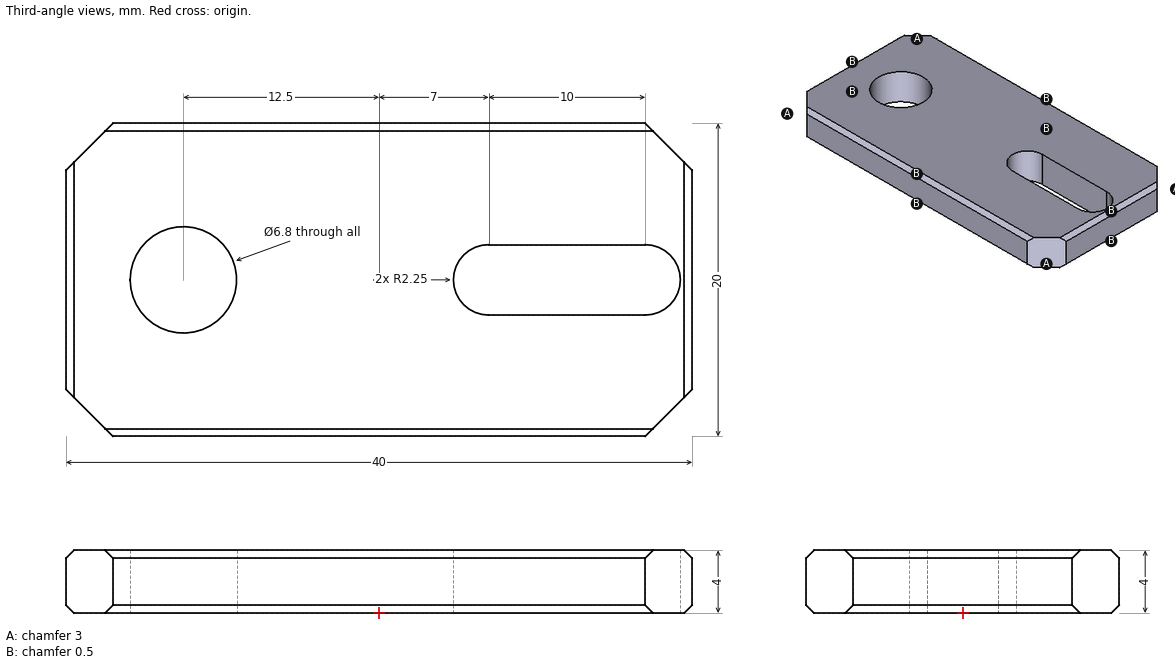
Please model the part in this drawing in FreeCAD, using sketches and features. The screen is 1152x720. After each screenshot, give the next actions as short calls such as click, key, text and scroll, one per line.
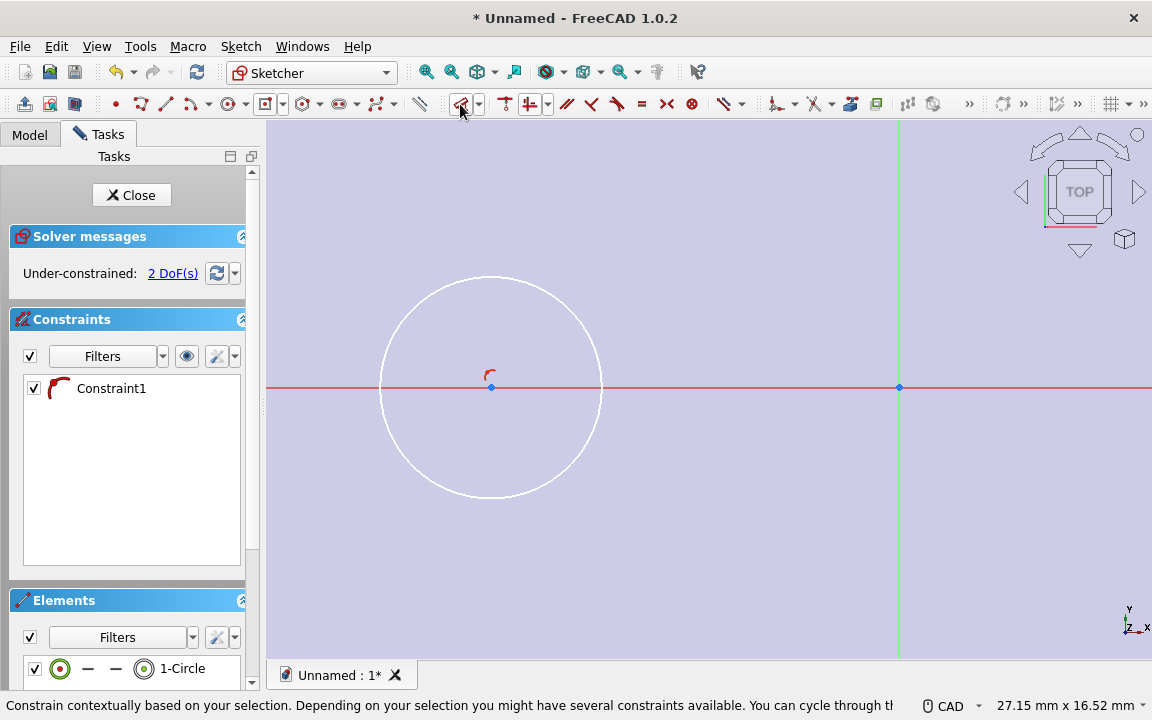
click(569, 309)
click(592, 286)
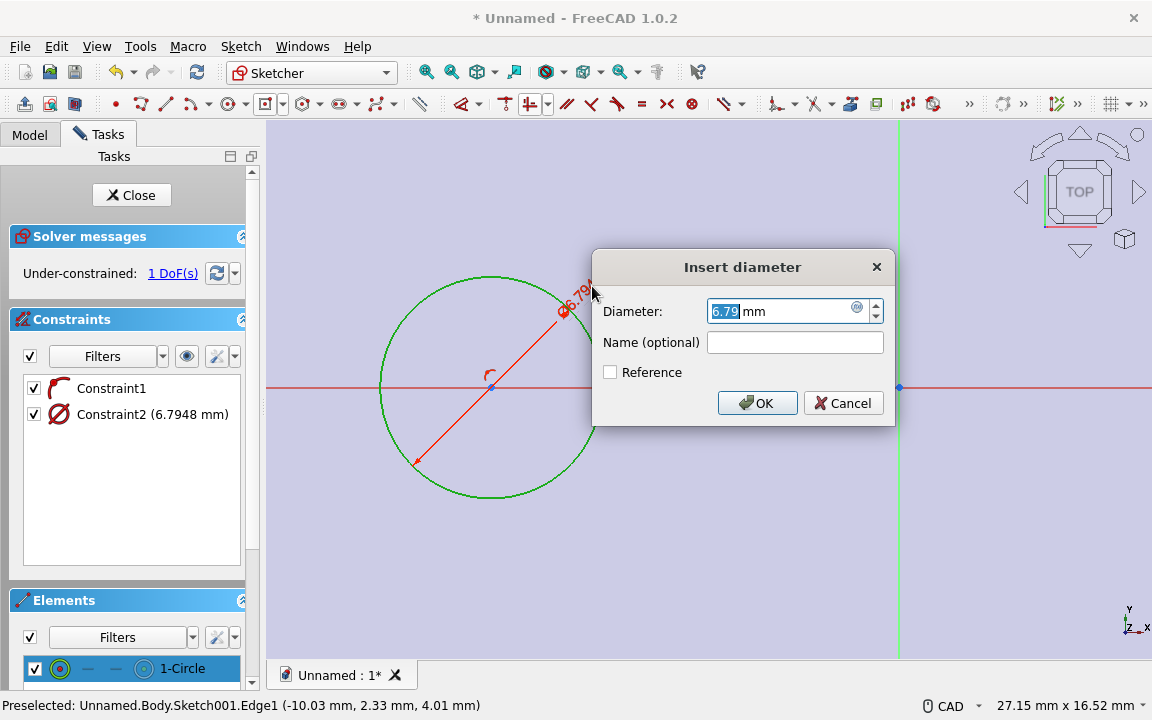
text(6.8)
key(Return)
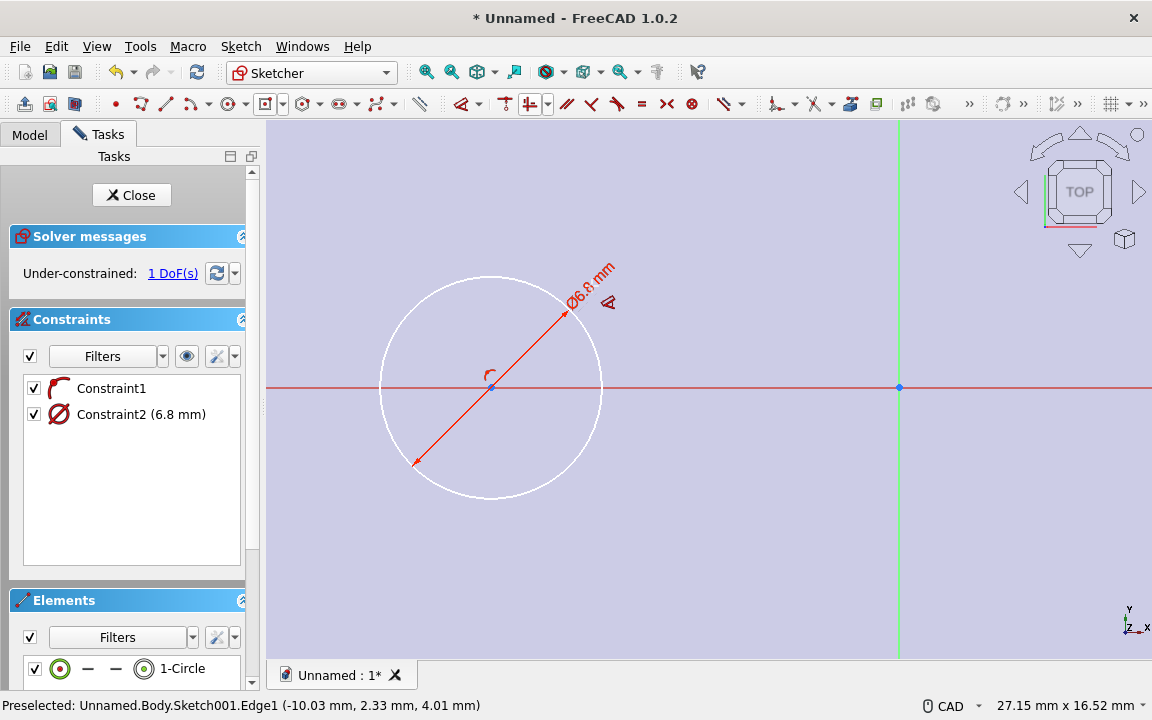
click(491, 388)
click(695, 422)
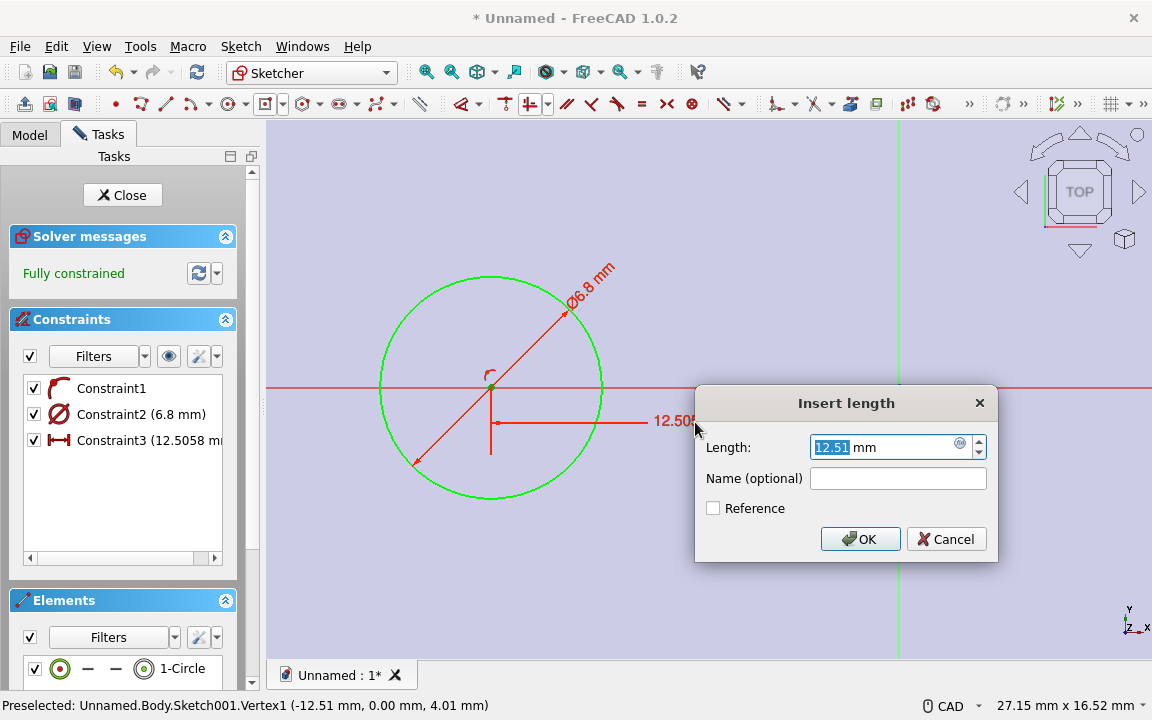
text(12.5)
key(Return)
key(Escape)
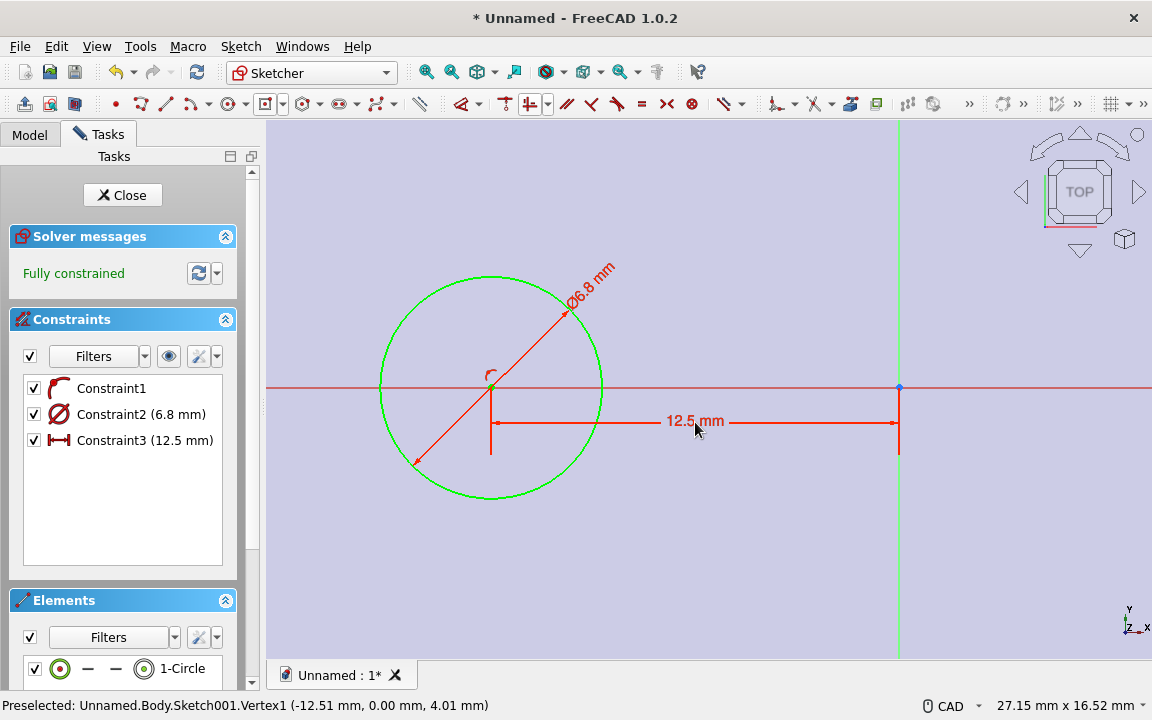
click(123, 195)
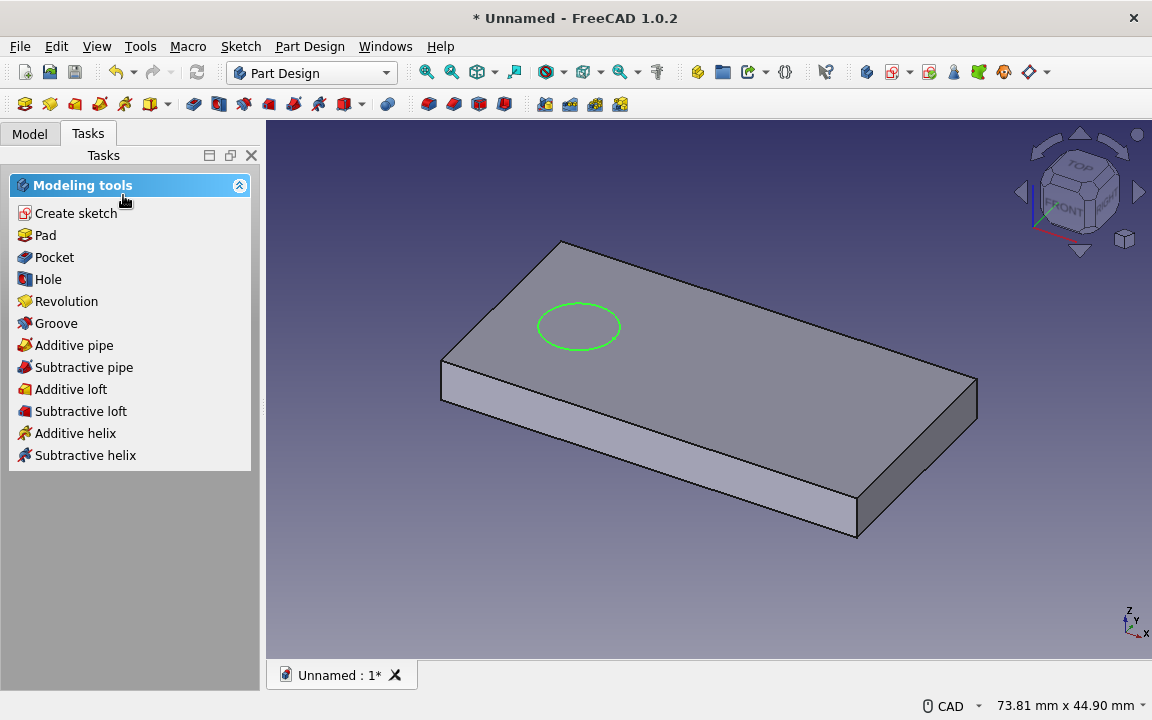
click(219, 104)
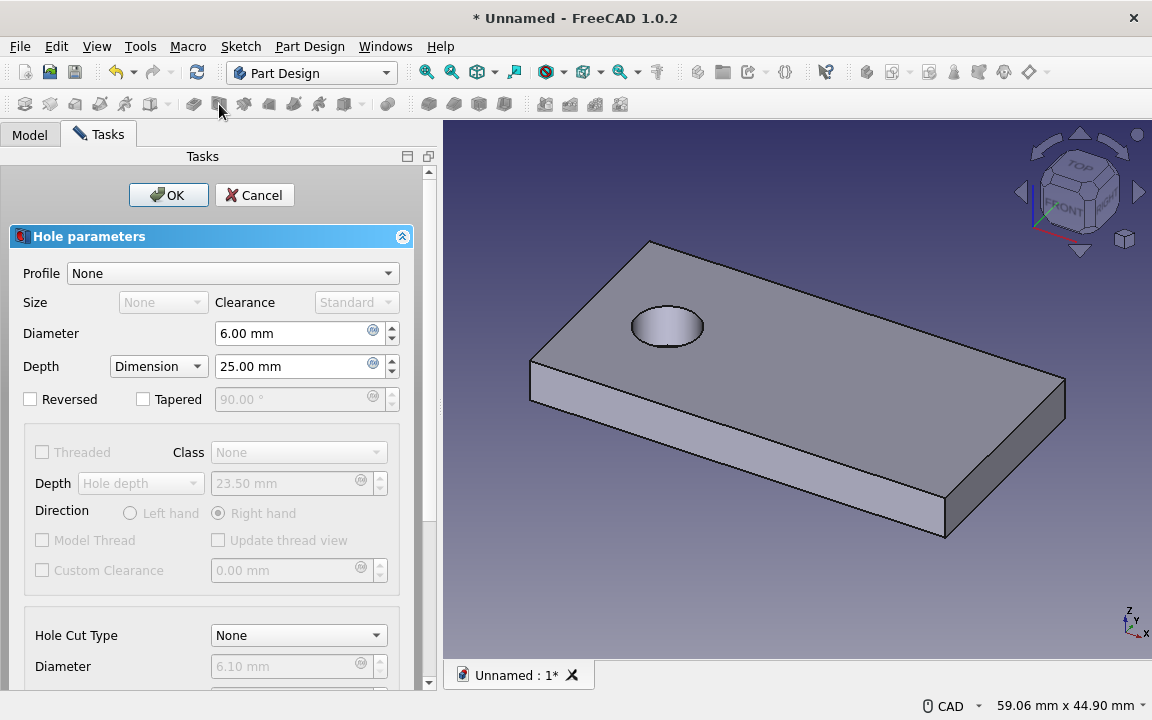
triple_click(300, 334)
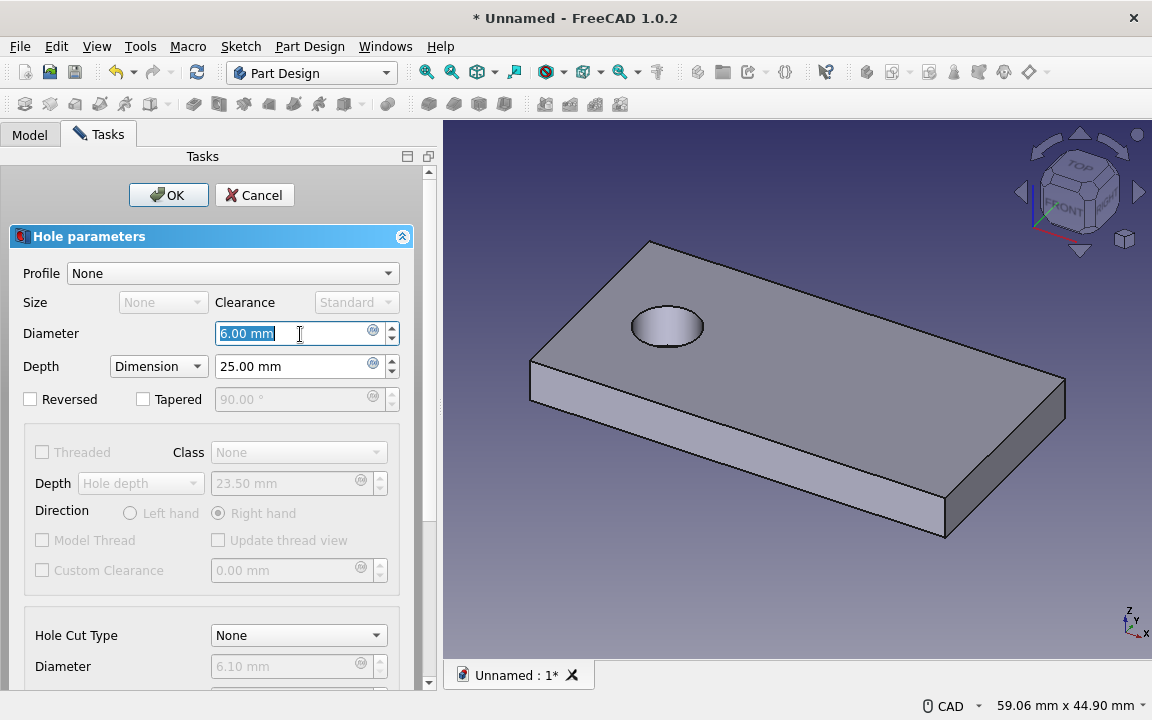
text(6.8)
key(Tab)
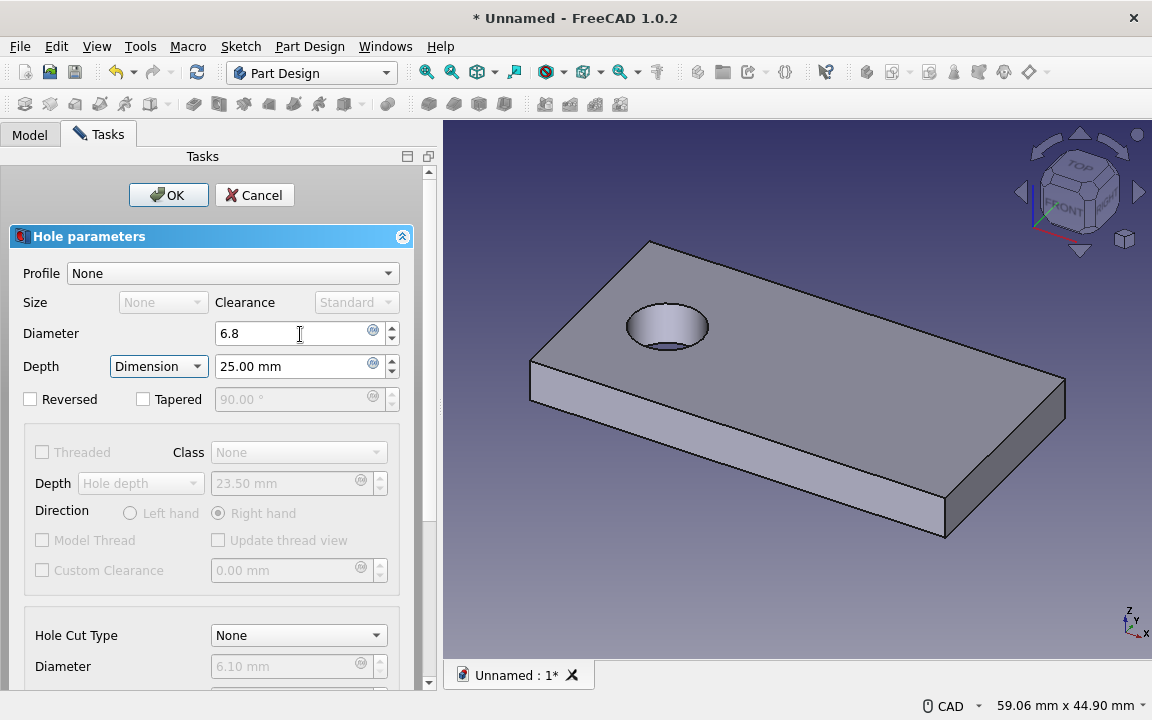
click(160, 366)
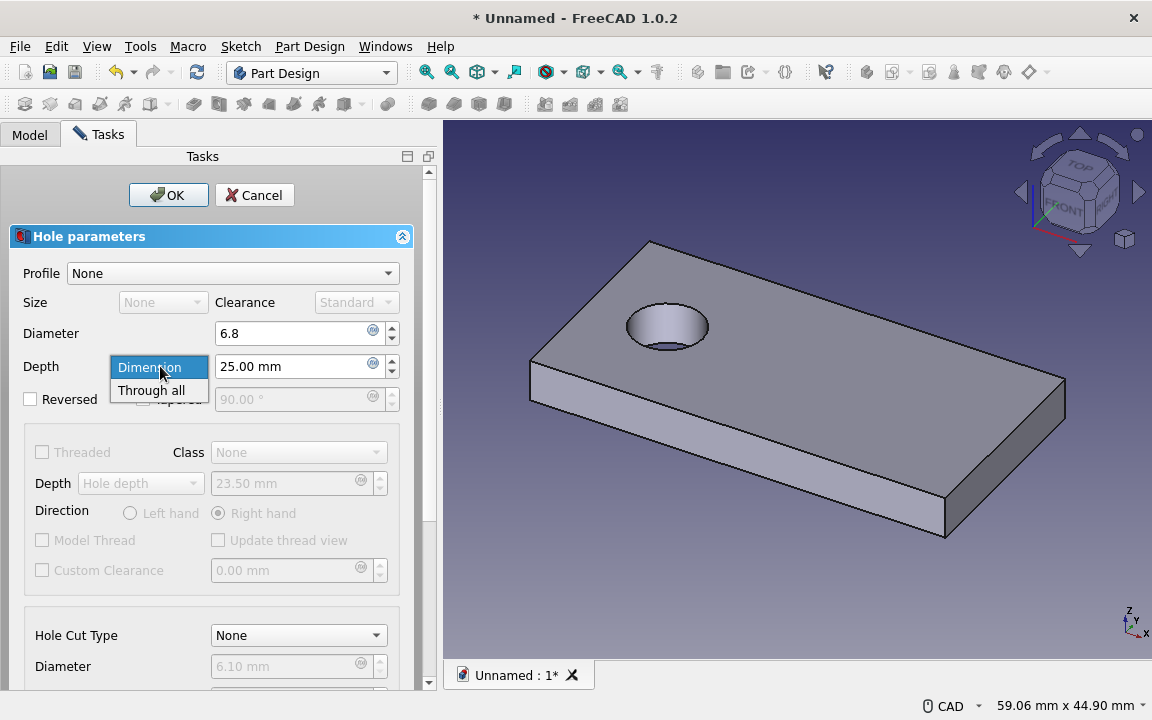
click(158, 390)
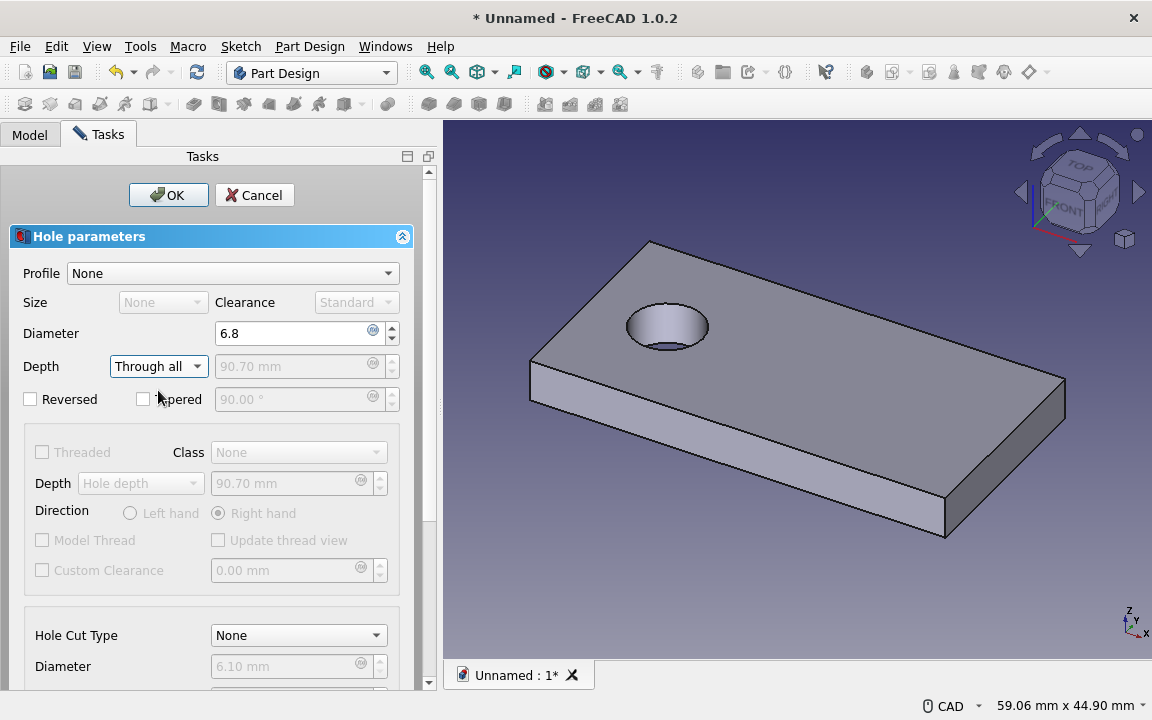
click(169, 195)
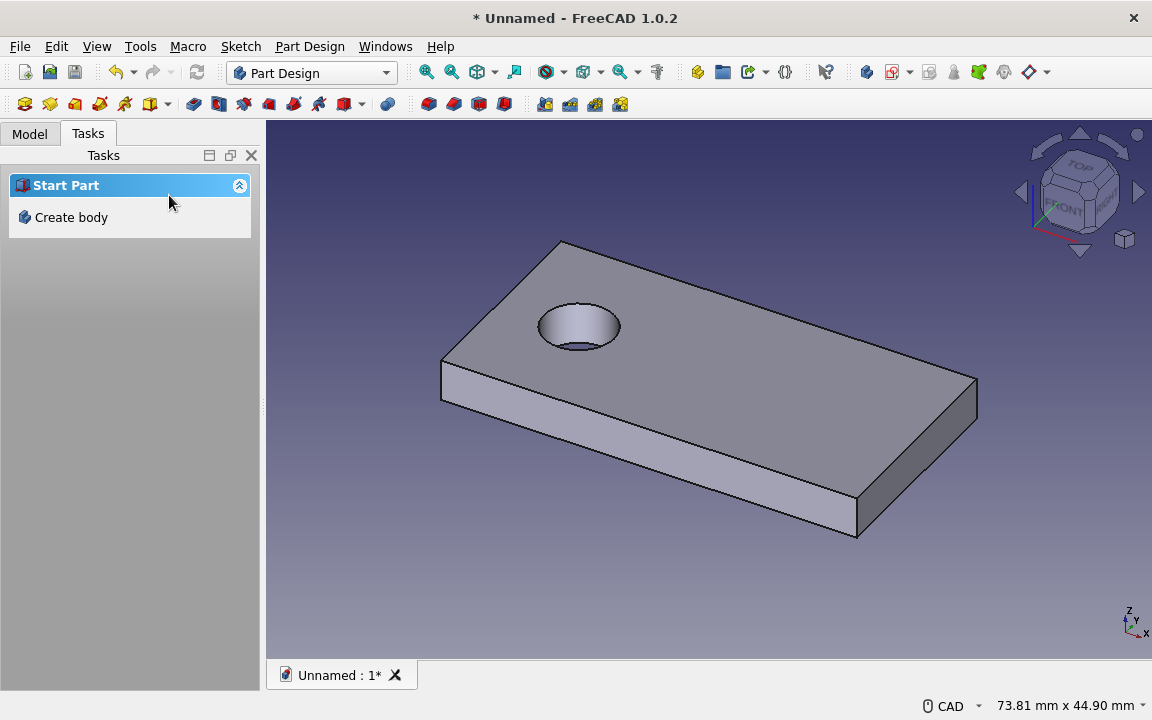
click(768, 389)